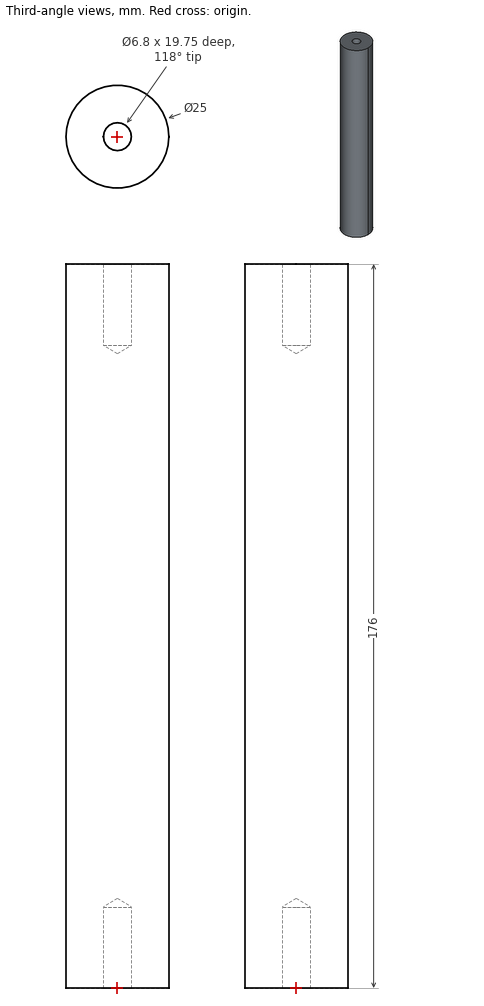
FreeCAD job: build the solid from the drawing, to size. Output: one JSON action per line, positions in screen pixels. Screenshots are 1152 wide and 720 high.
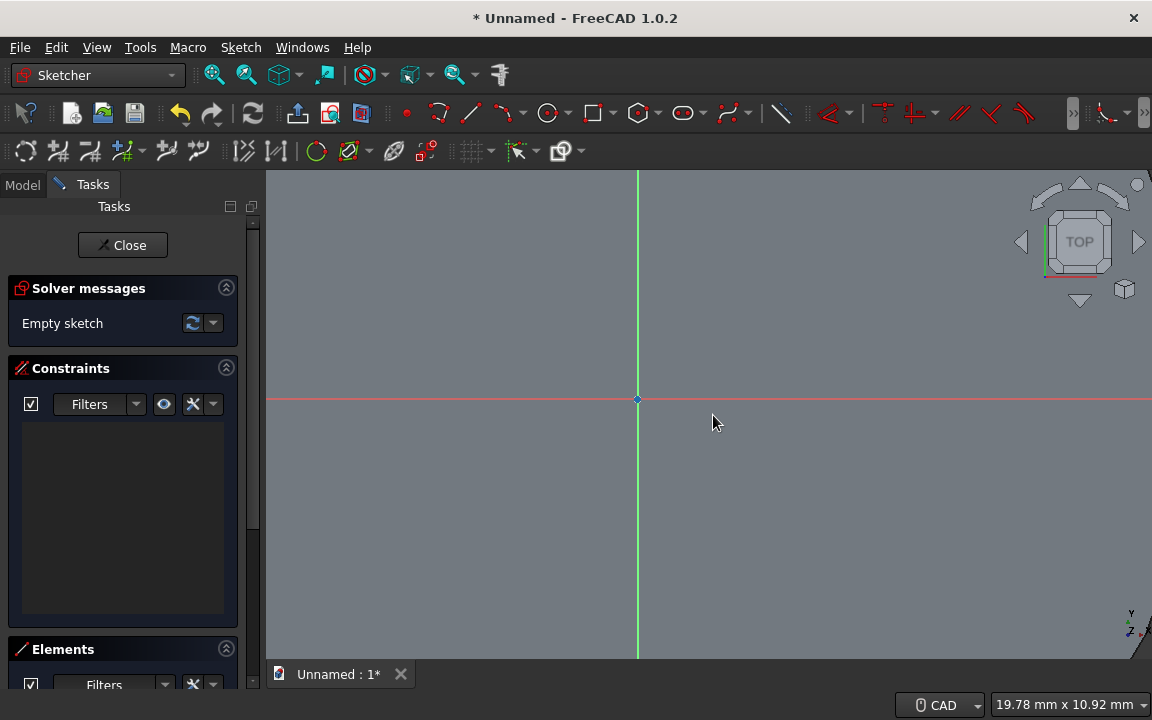
{"action": "left_click", "coordinate": [548, 114]}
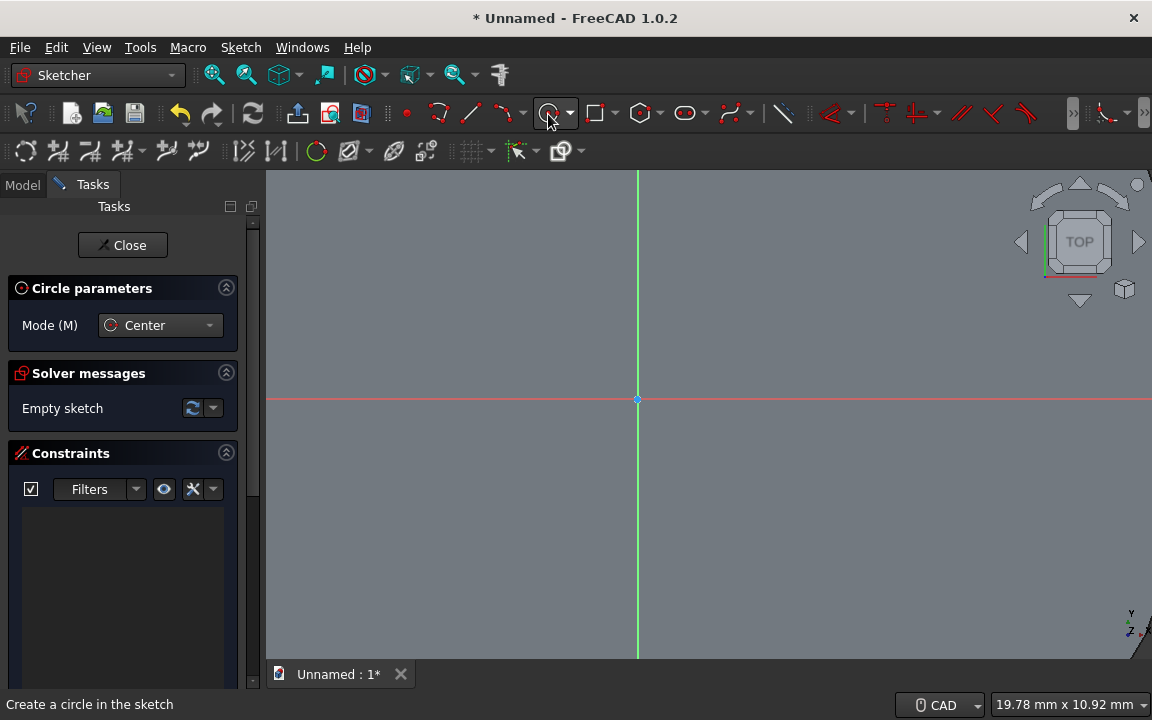
{"action": "left_click", "coordinate": [638, 399]}
{"action": "left_click", "coordinate": [745, 291]}
{"action": "key", "text": "Escape"}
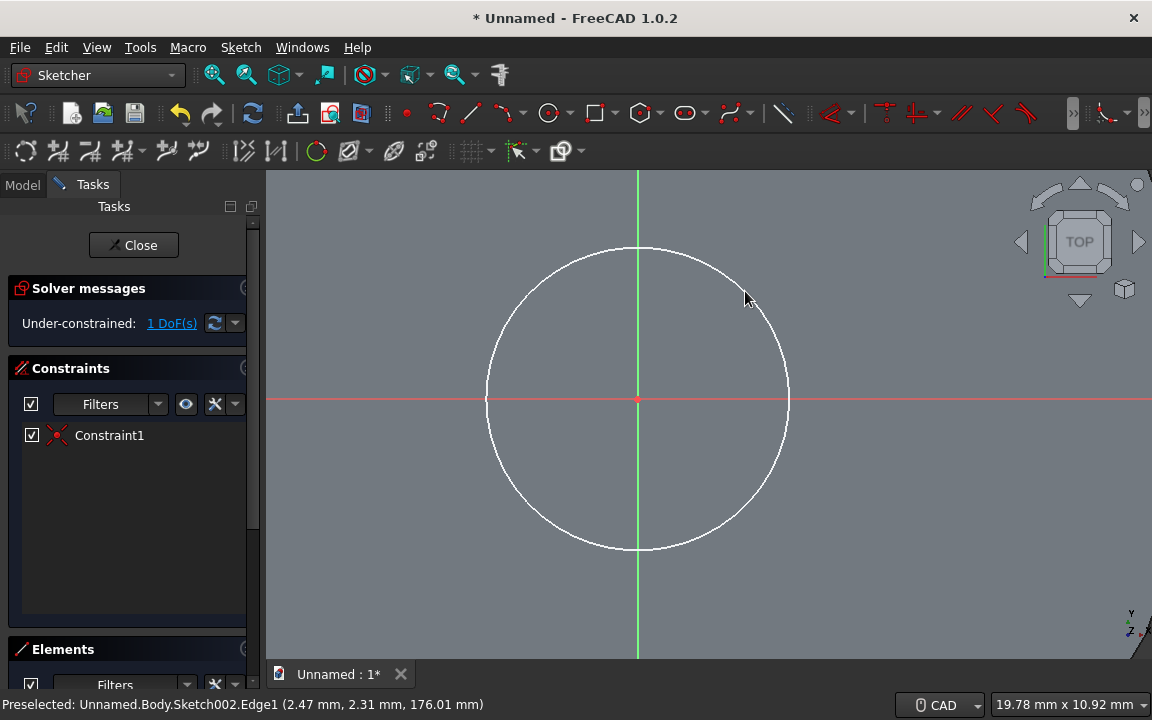
{"action": "left_click", "coordinate": [830, 114]}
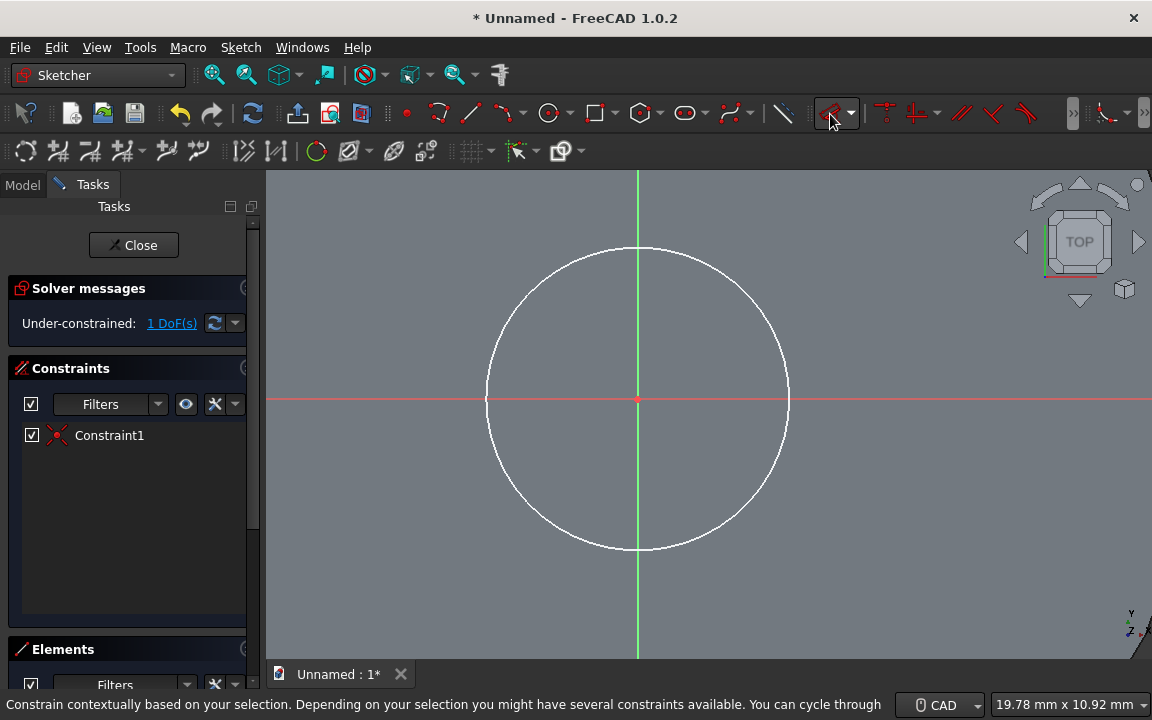
{"action": "left_click", "coordinate": [745, 292]}
{"action": "left_click", "coordinate": [768, 269]}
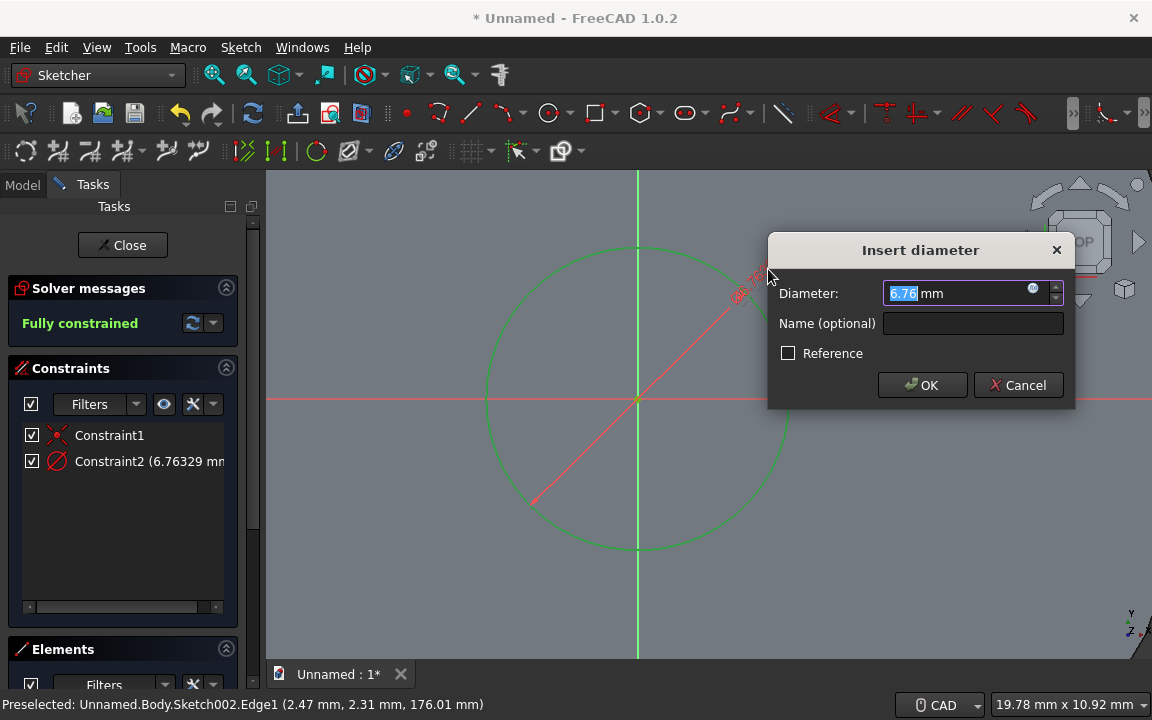
{"action": "type", "text": "6.8"}
{"action": "key", "text": "Return"}
{"action": "key", "text": "Escape"}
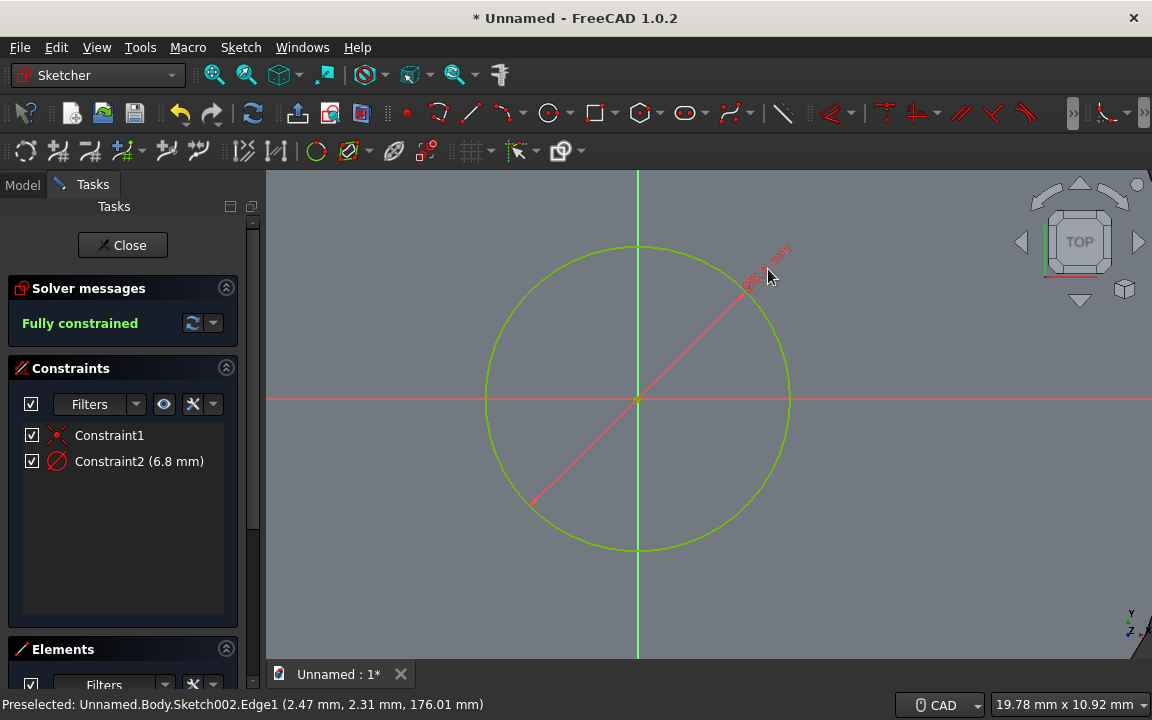
{"action": "left_click", "coordinate": [123, 245]}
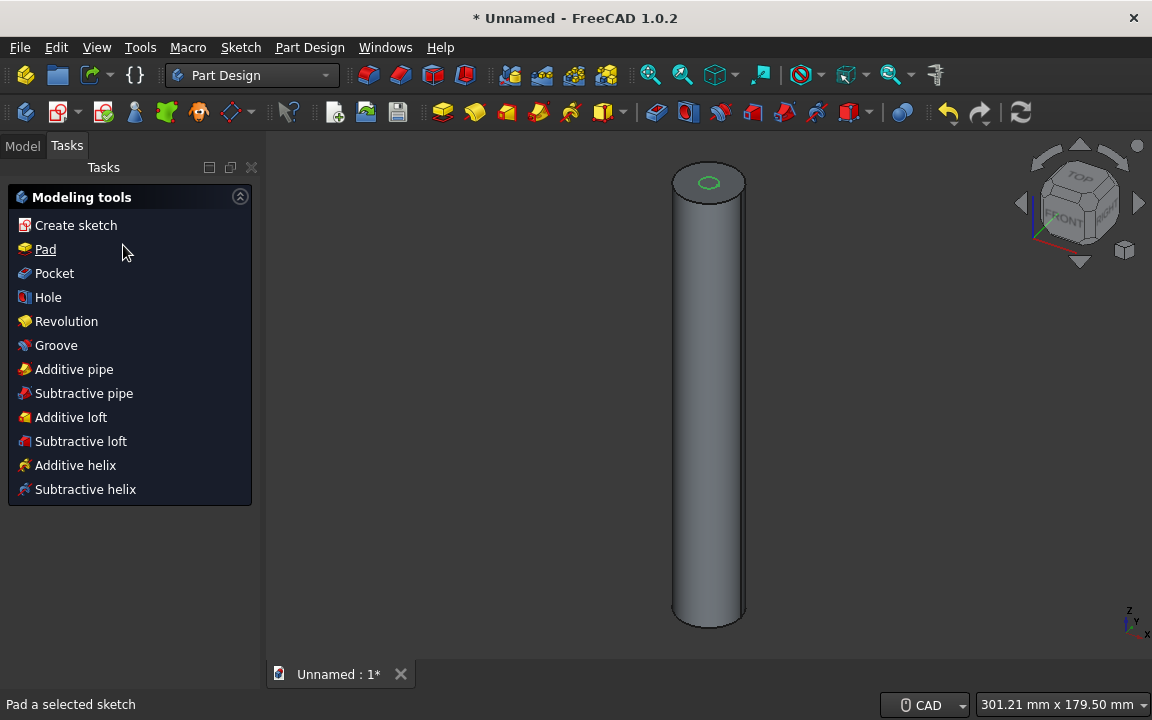
{"action": "left_click", "coordinate": [690, 112]}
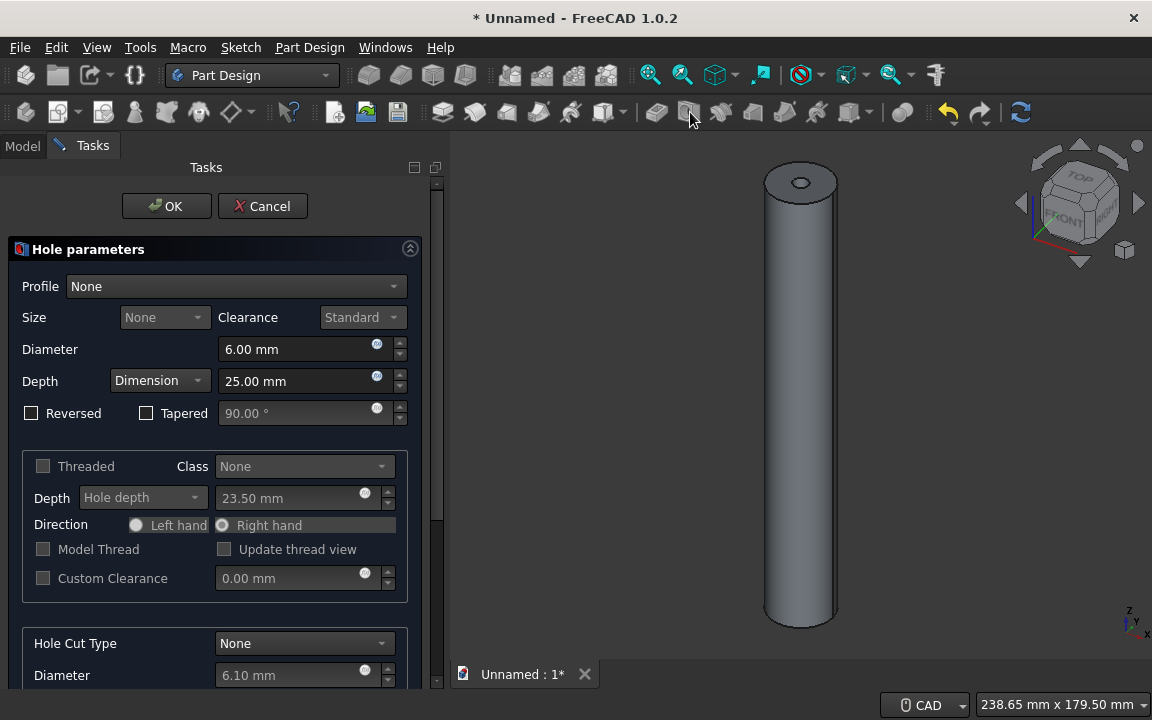
{"action": "triple_click", "coordinate": [305, 349]}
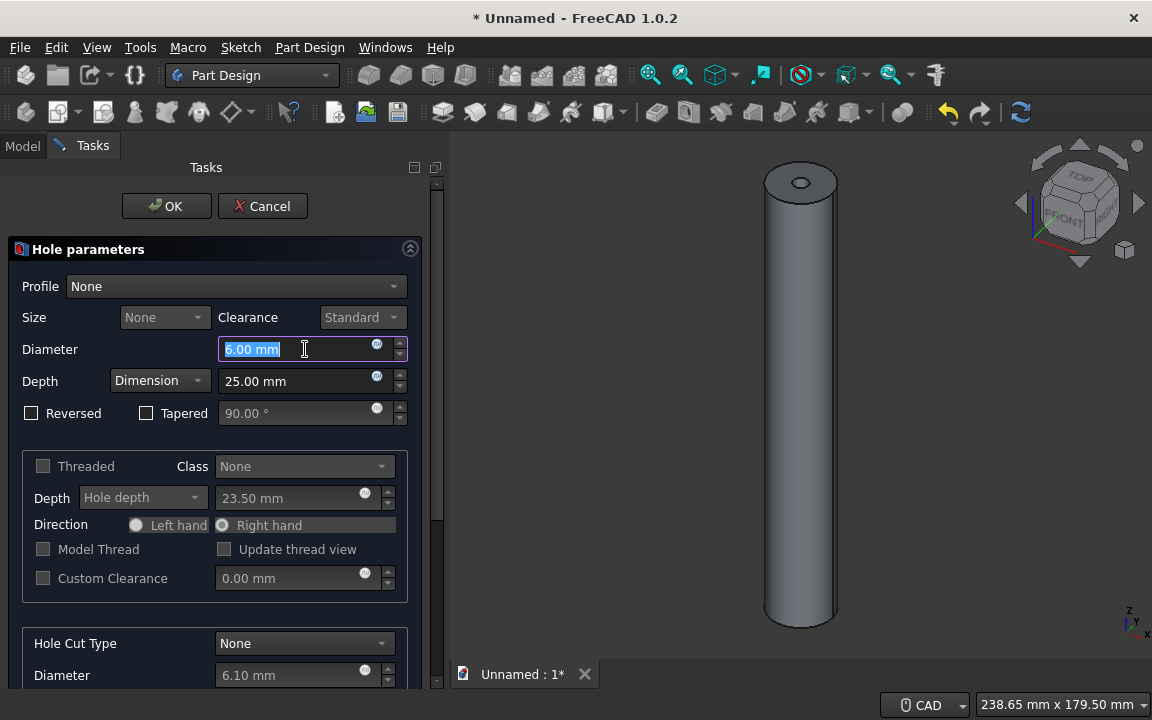
{"action": "type", "text": "6.8"}
{"action": "key", "text": "Tab"}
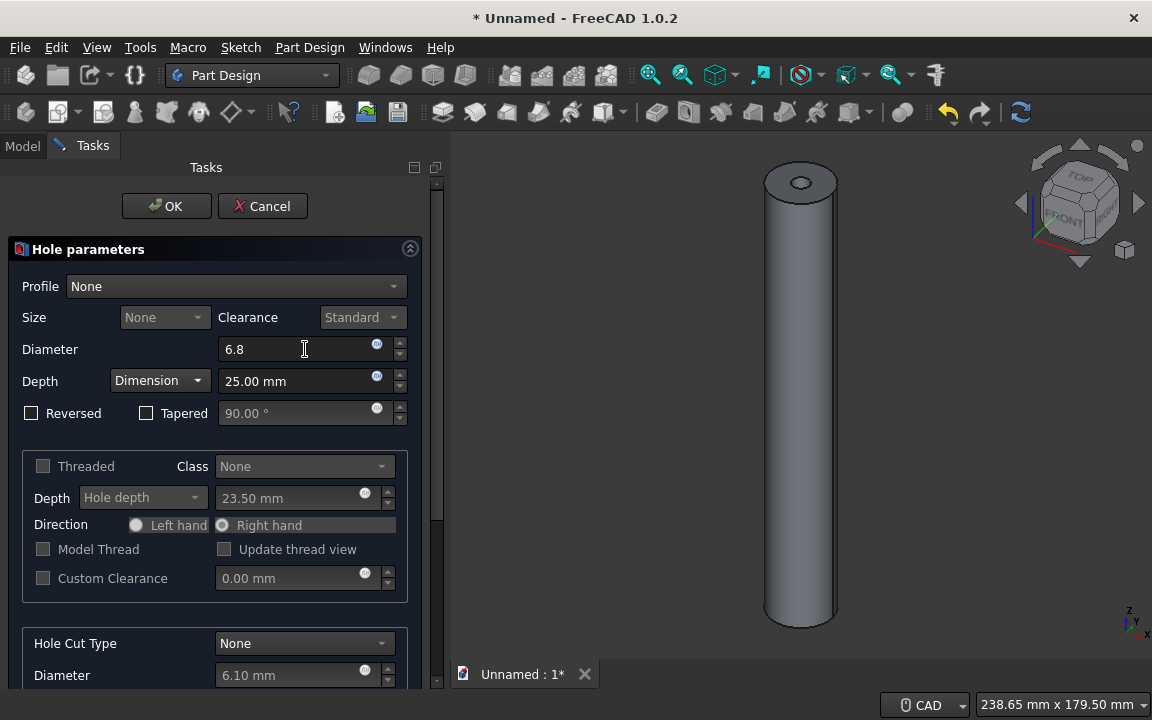
{"action": "triple_click", "coordinate": [305, 381]}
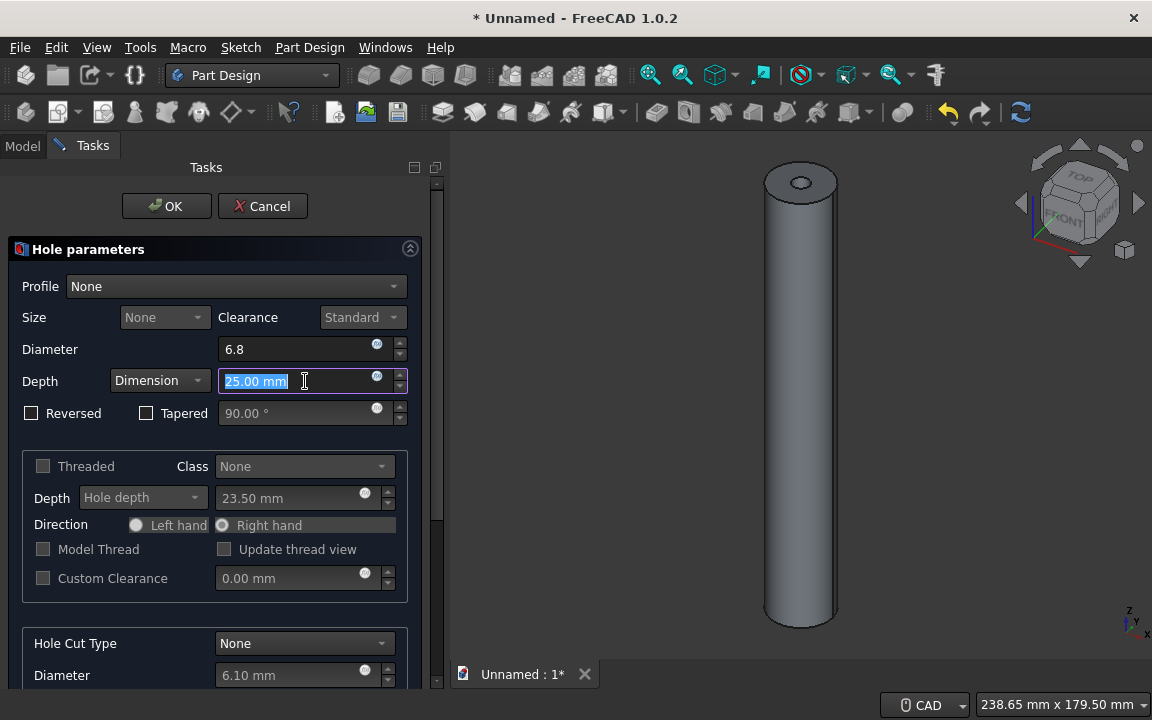
{"action": "type", "text": "19.75"}
{"action": "key", "text": "Tab"}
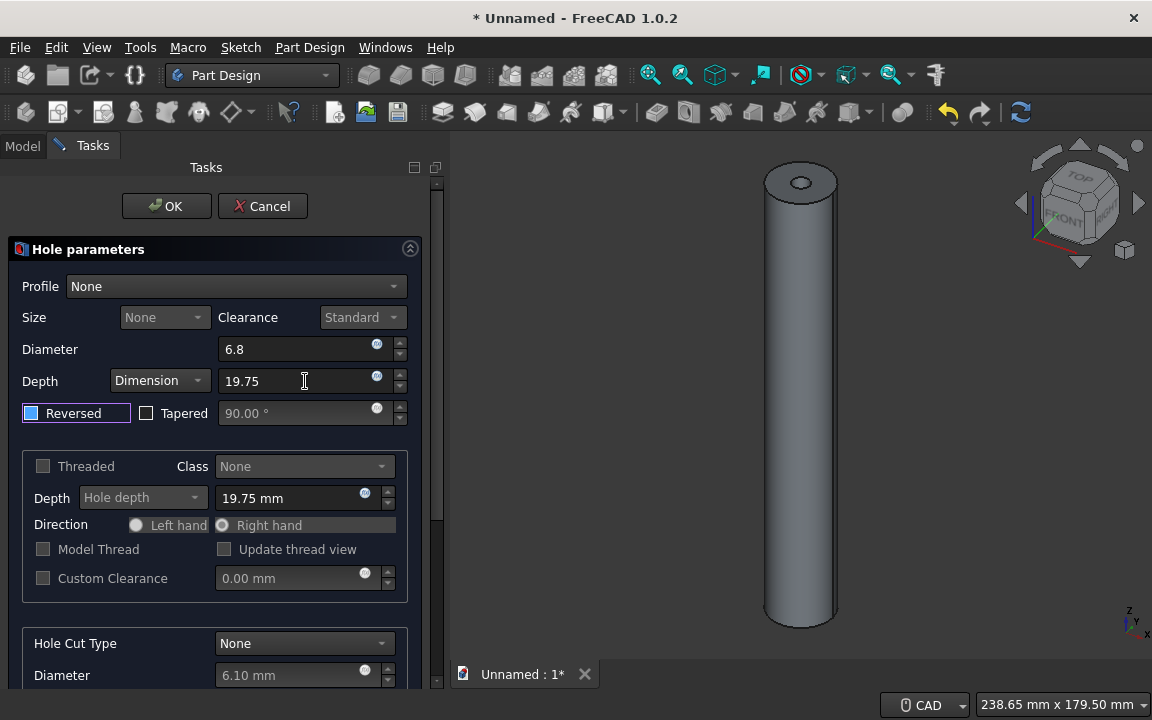
{"action": "left_click", "coordinate": [167, 206]}